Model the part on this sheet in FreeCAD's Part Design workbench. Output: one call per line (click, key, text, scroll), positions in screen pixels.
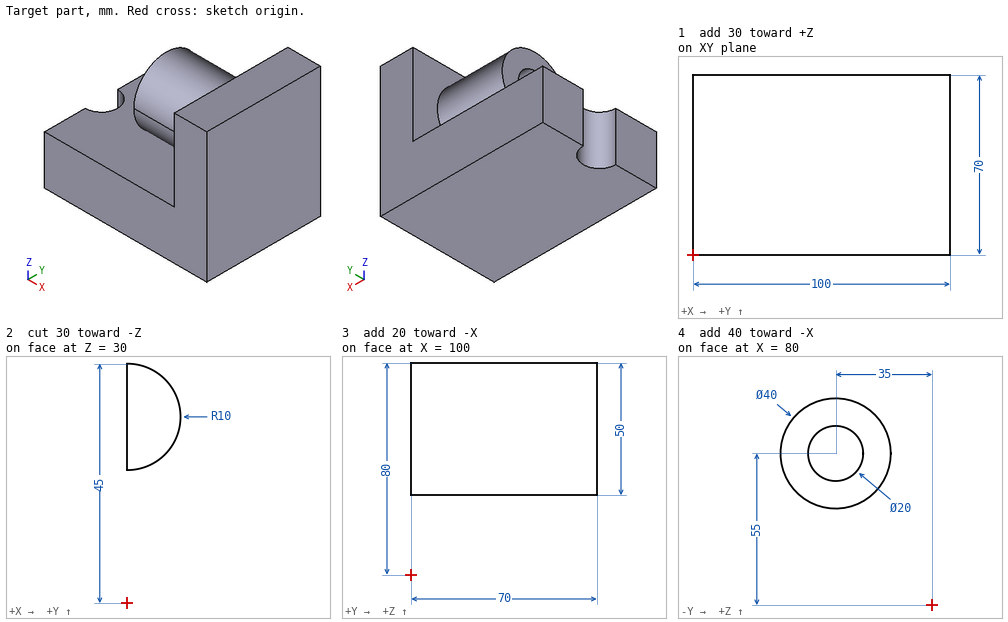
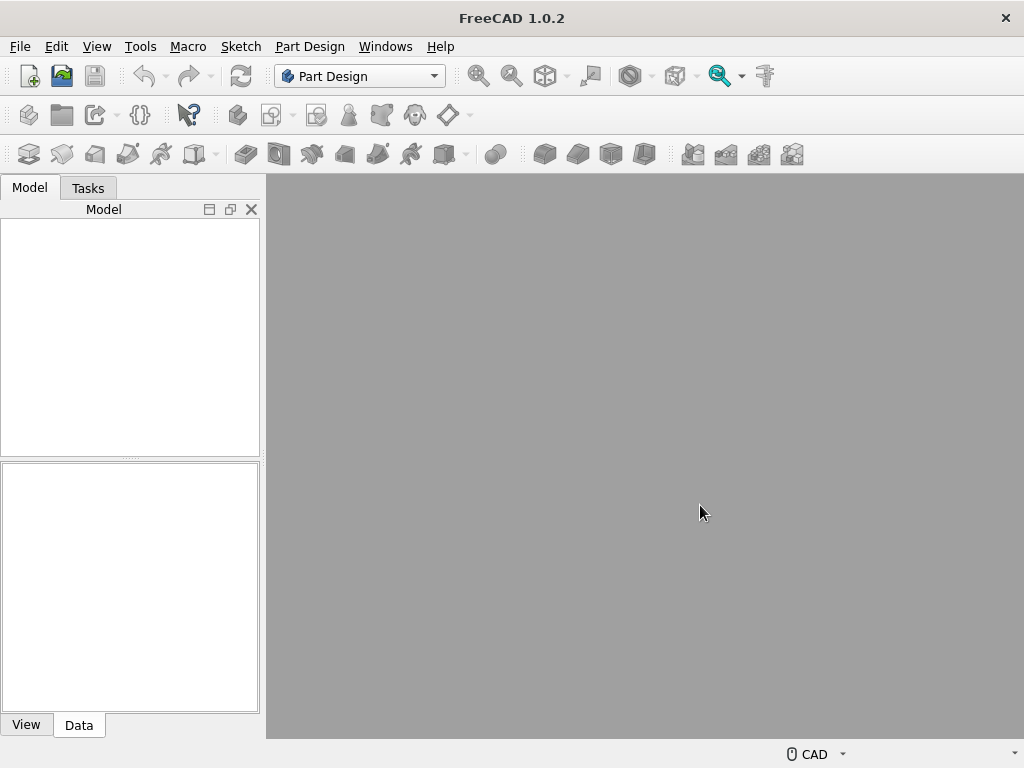
click(29, 76)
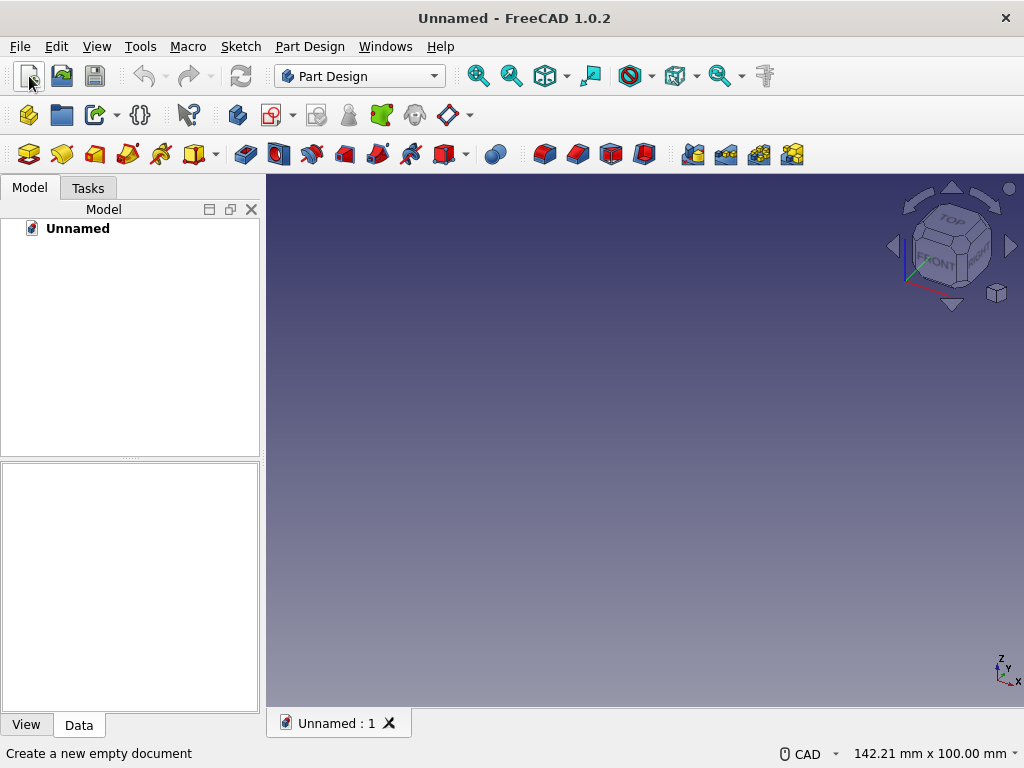
click(270, 116)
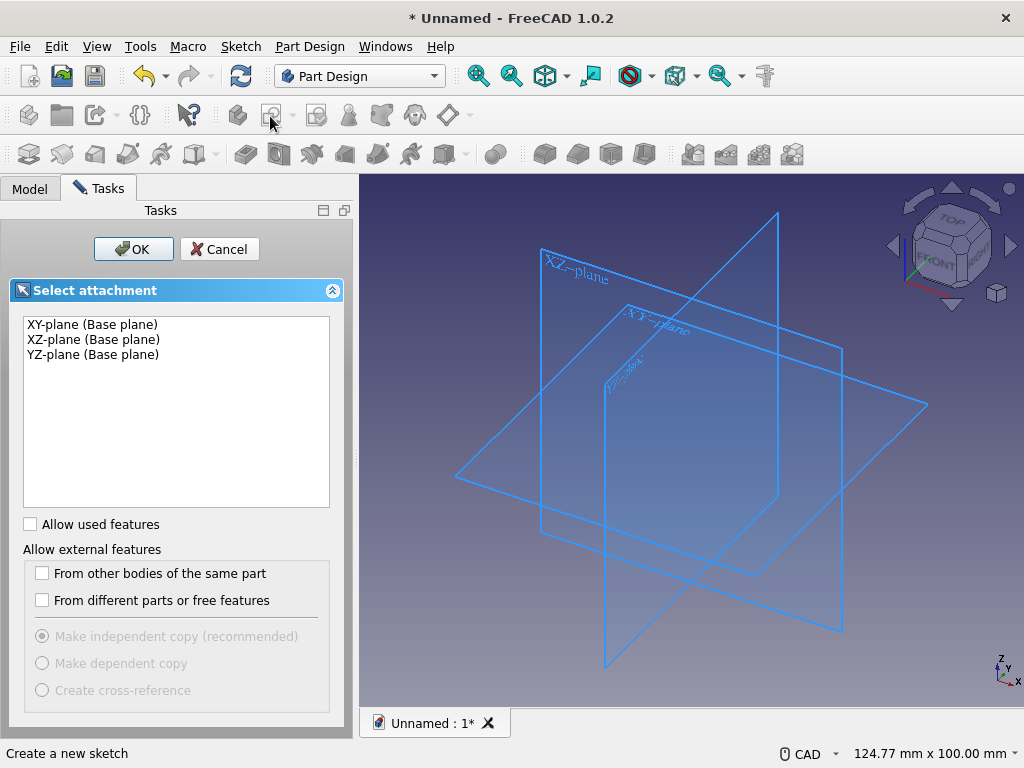
click(84, 324)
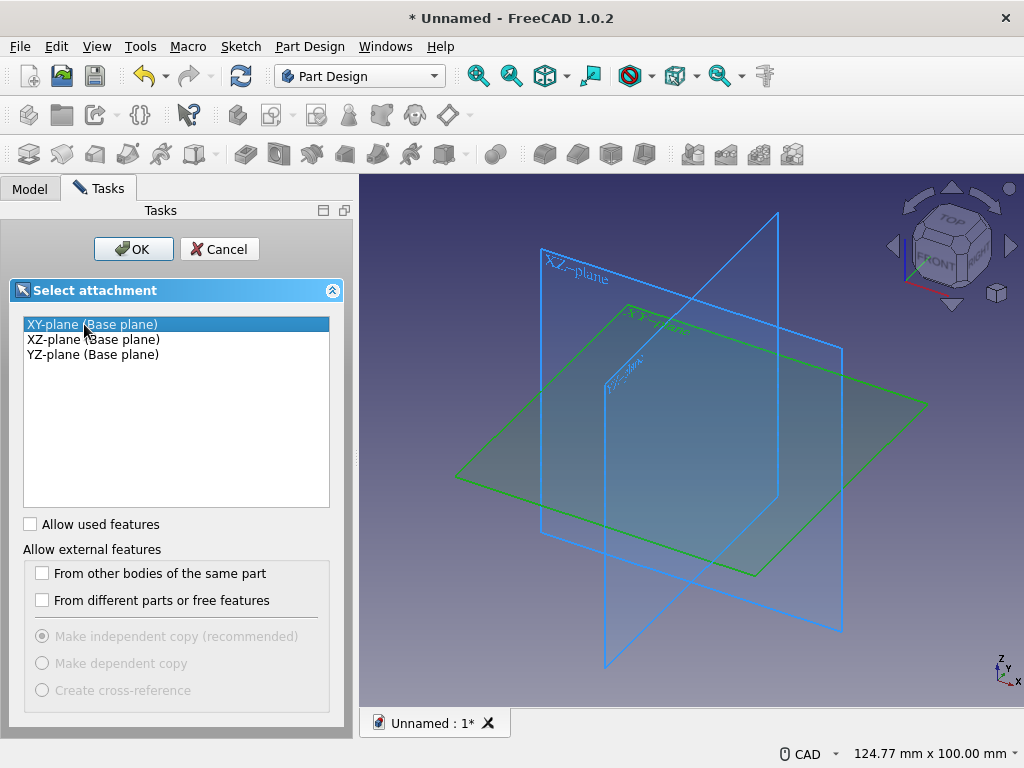
click(134, 249)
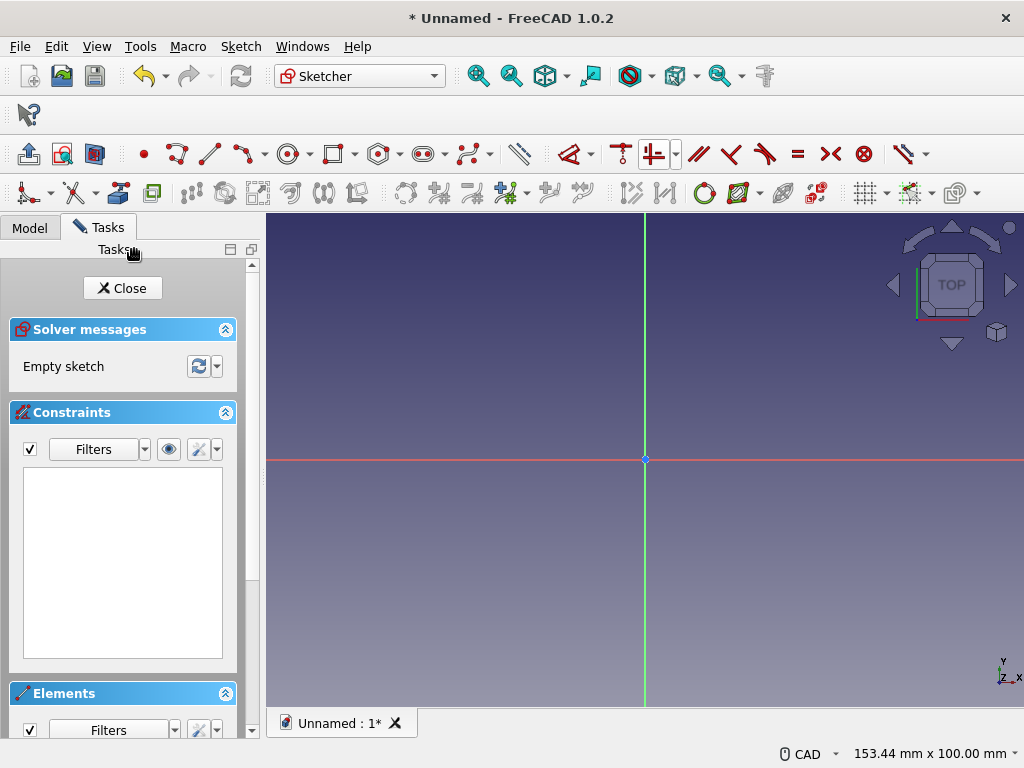
scroll(294, 670, down, 3)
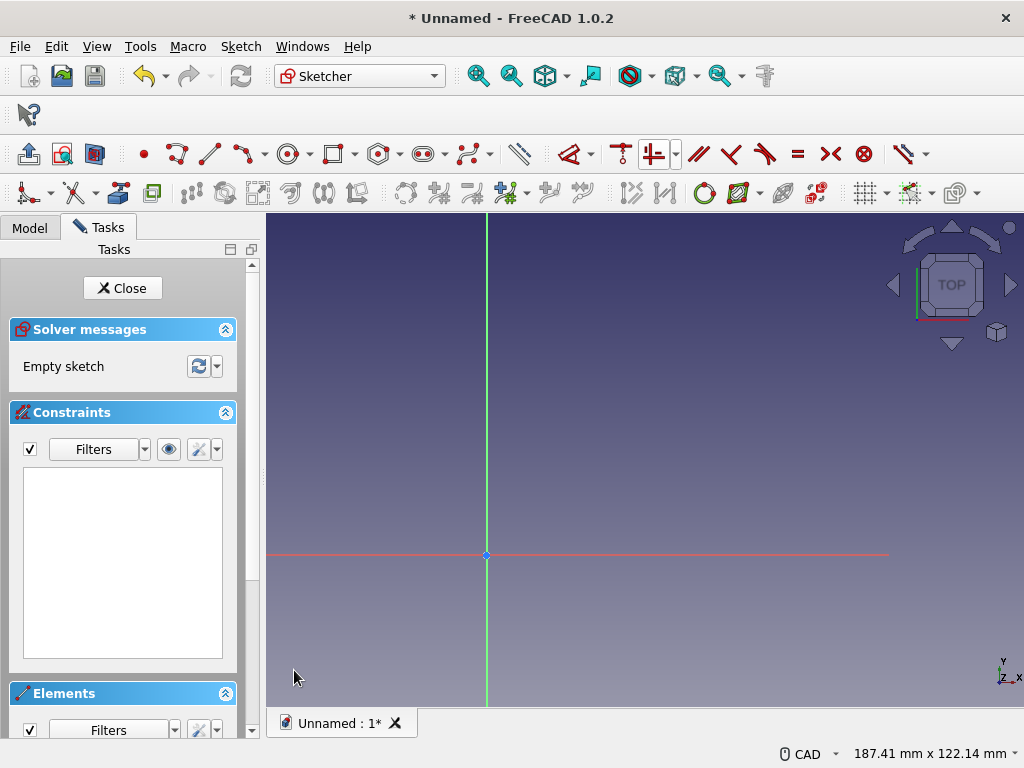
scroll(715, 461, up, 2)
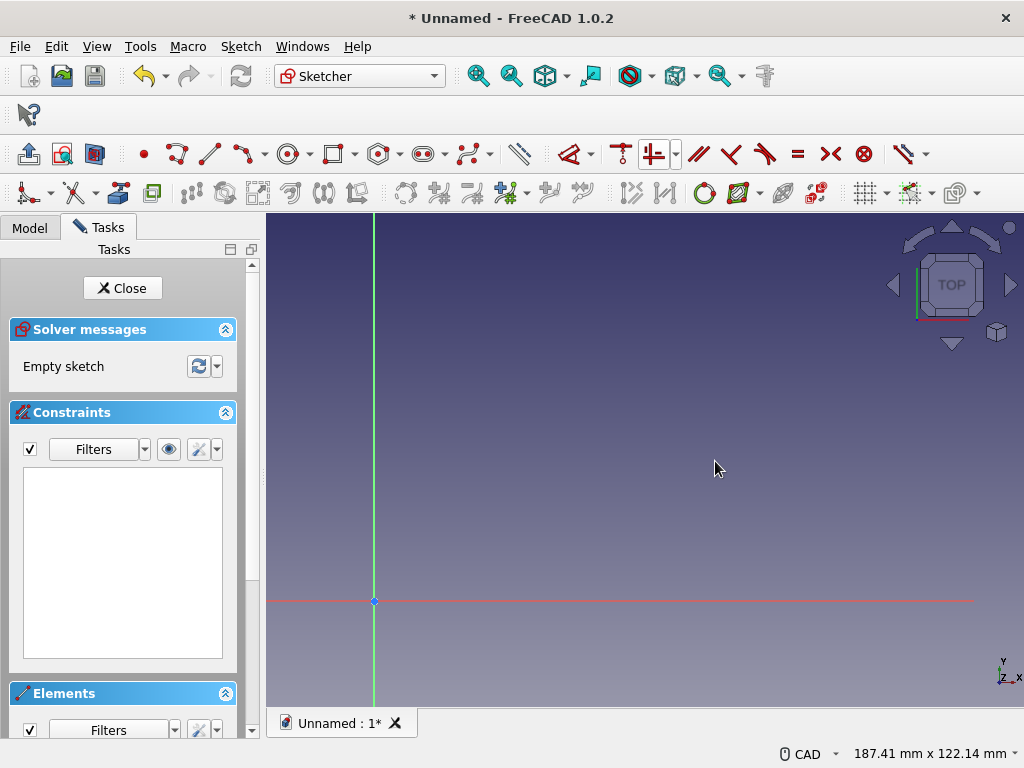
click(332, 154)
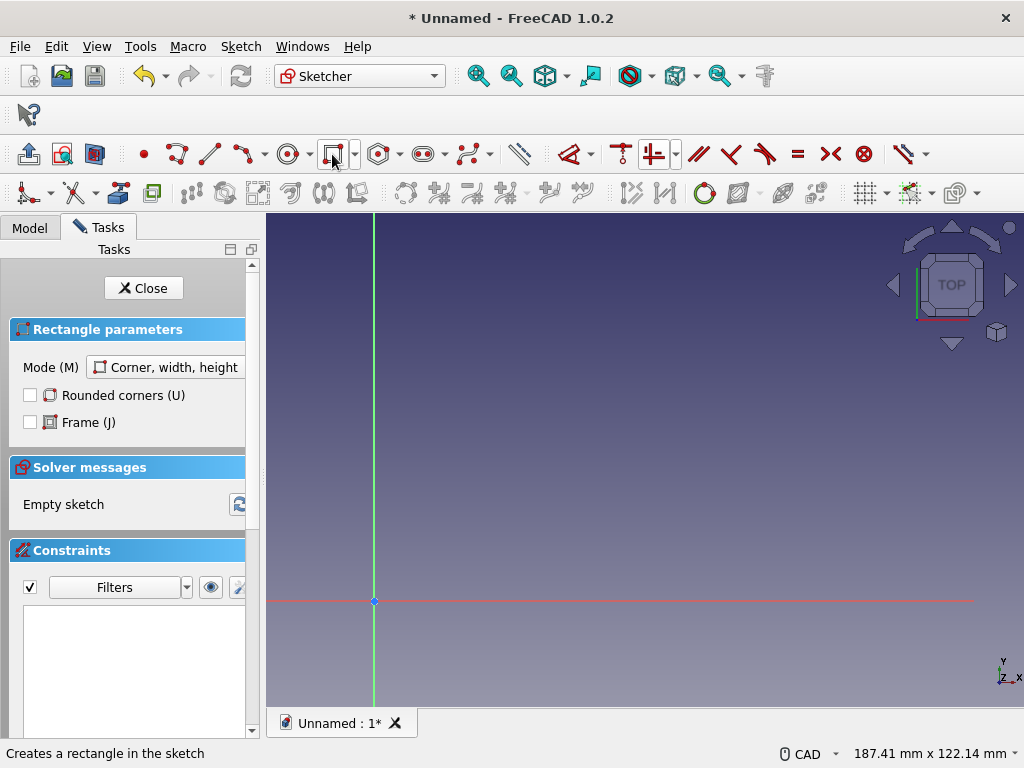
click(374, 601)
move(779, 318)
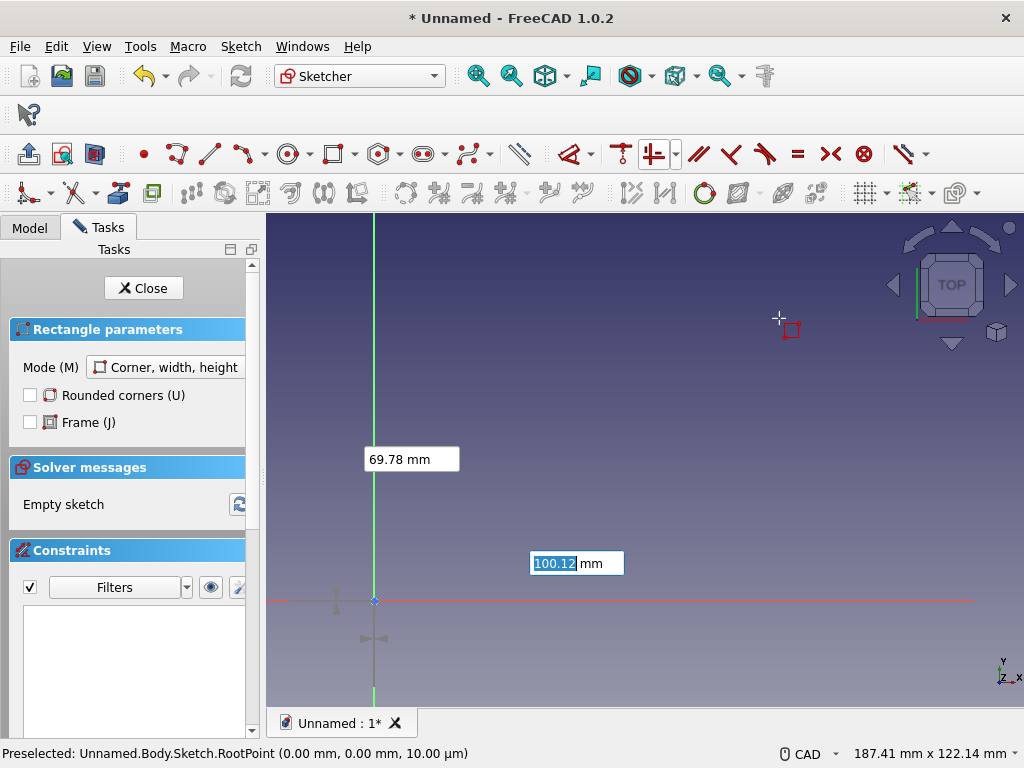
text(100)
key(Tab)
text(70)
key(Return)
key(Escape)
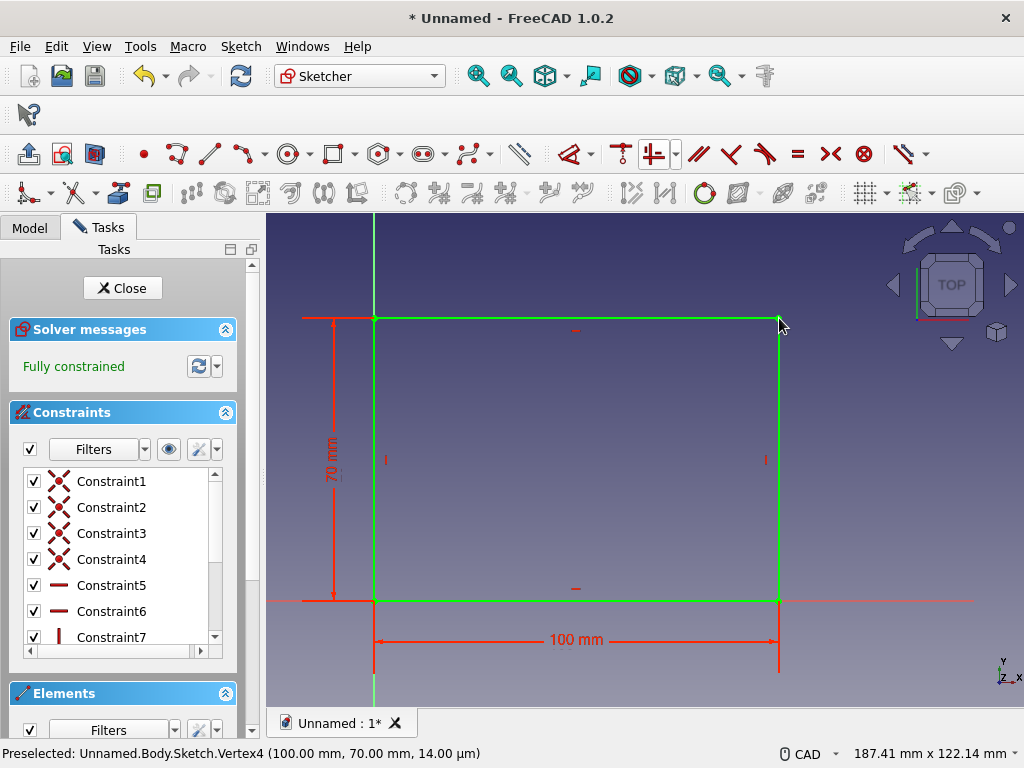
click(123, 288)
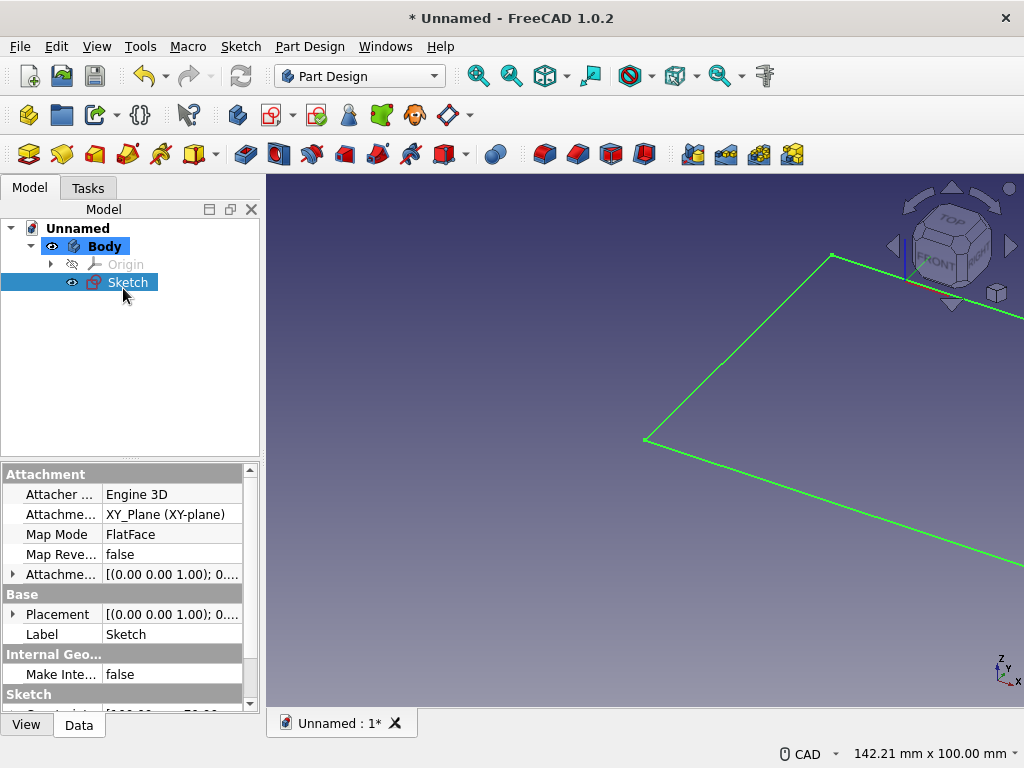
click(29, 154)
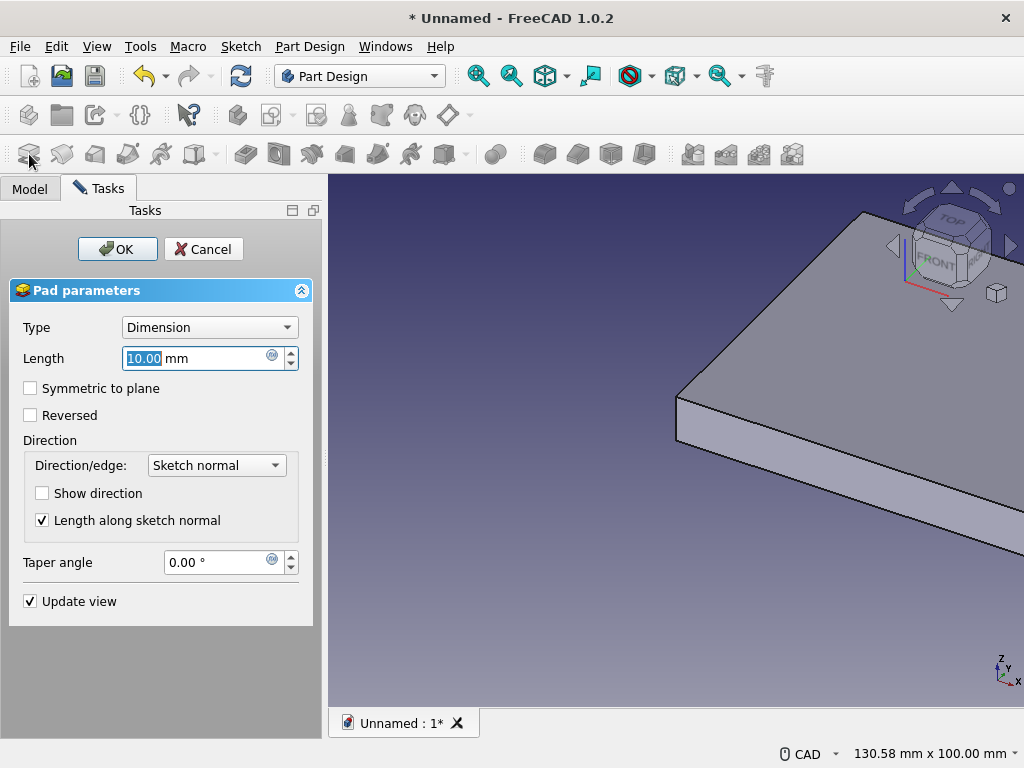
text(30)
key(Tab)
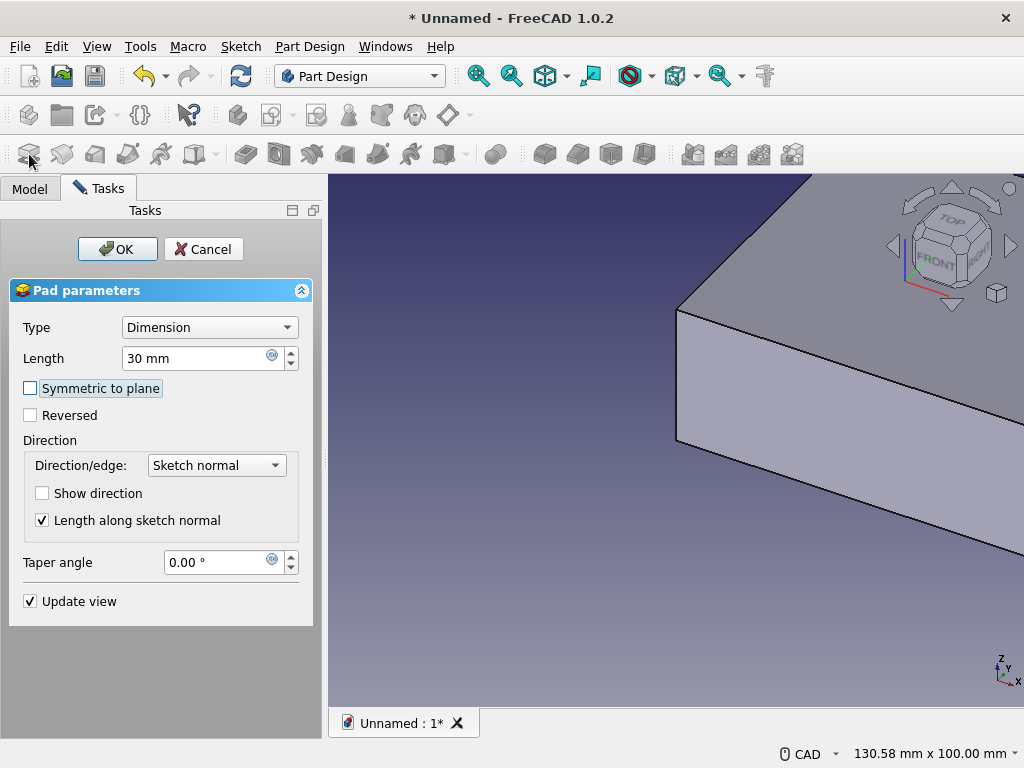
click(118, 249)